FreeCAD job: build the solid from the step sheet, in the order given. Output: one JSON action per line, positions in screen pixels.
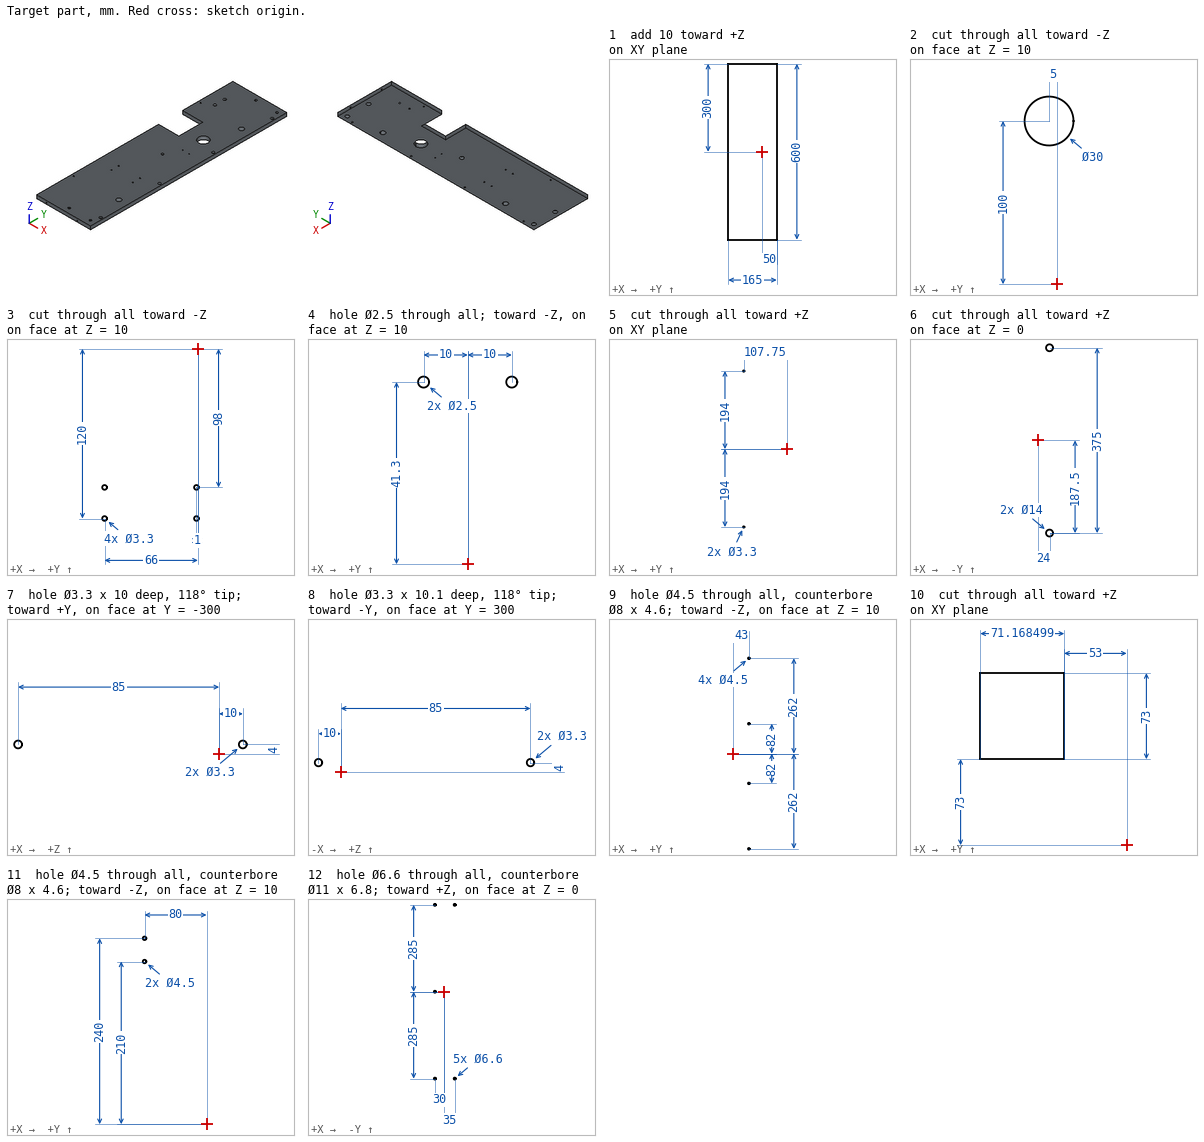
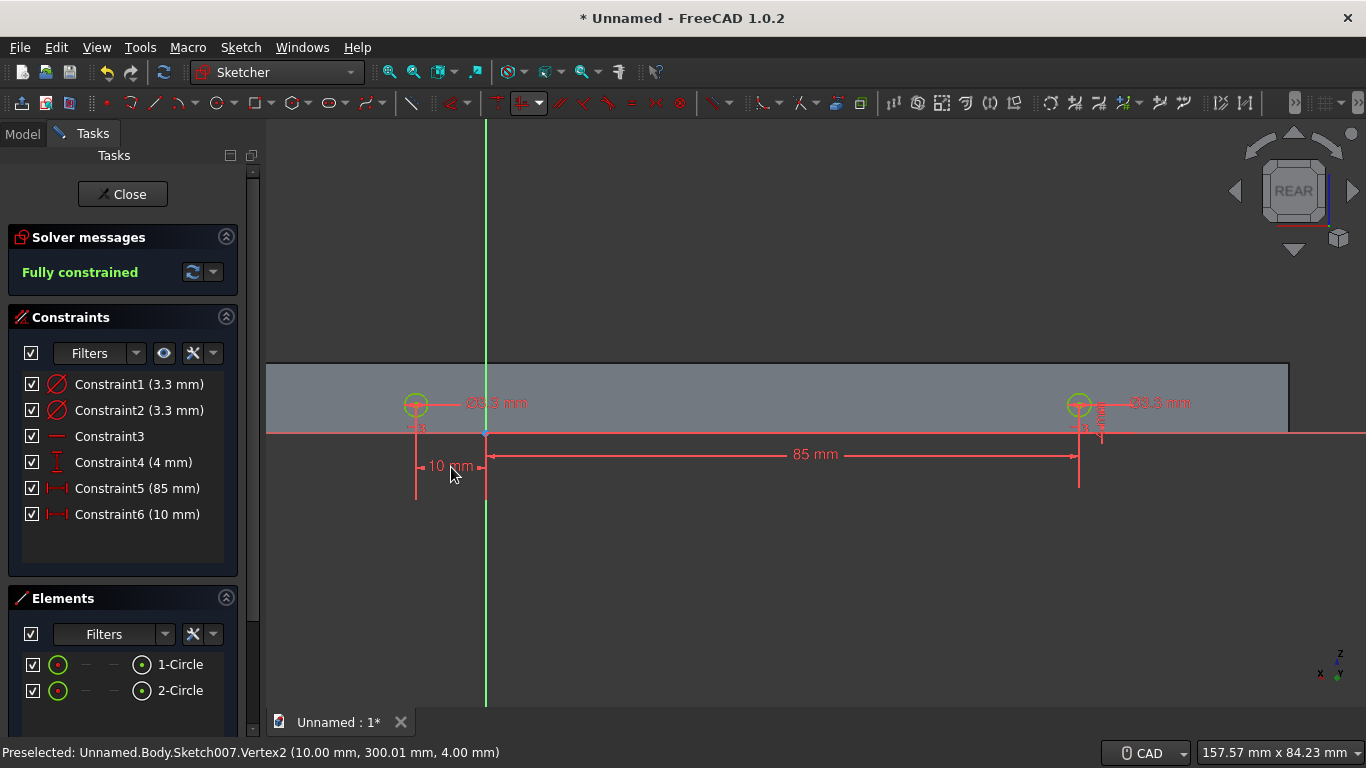
{"action": "left_click", "coordinate": [123, 194]}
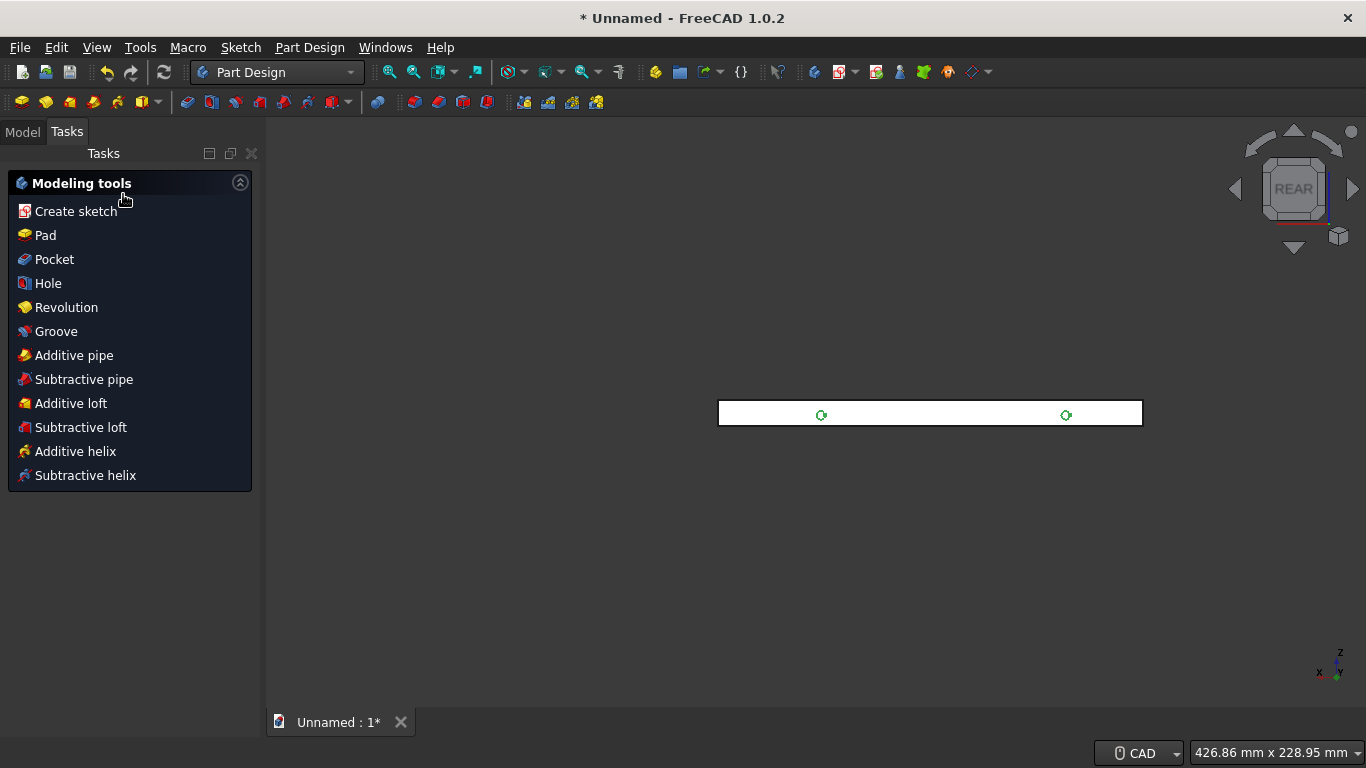
{"action": "left_click", "coordinate": [212, 102]}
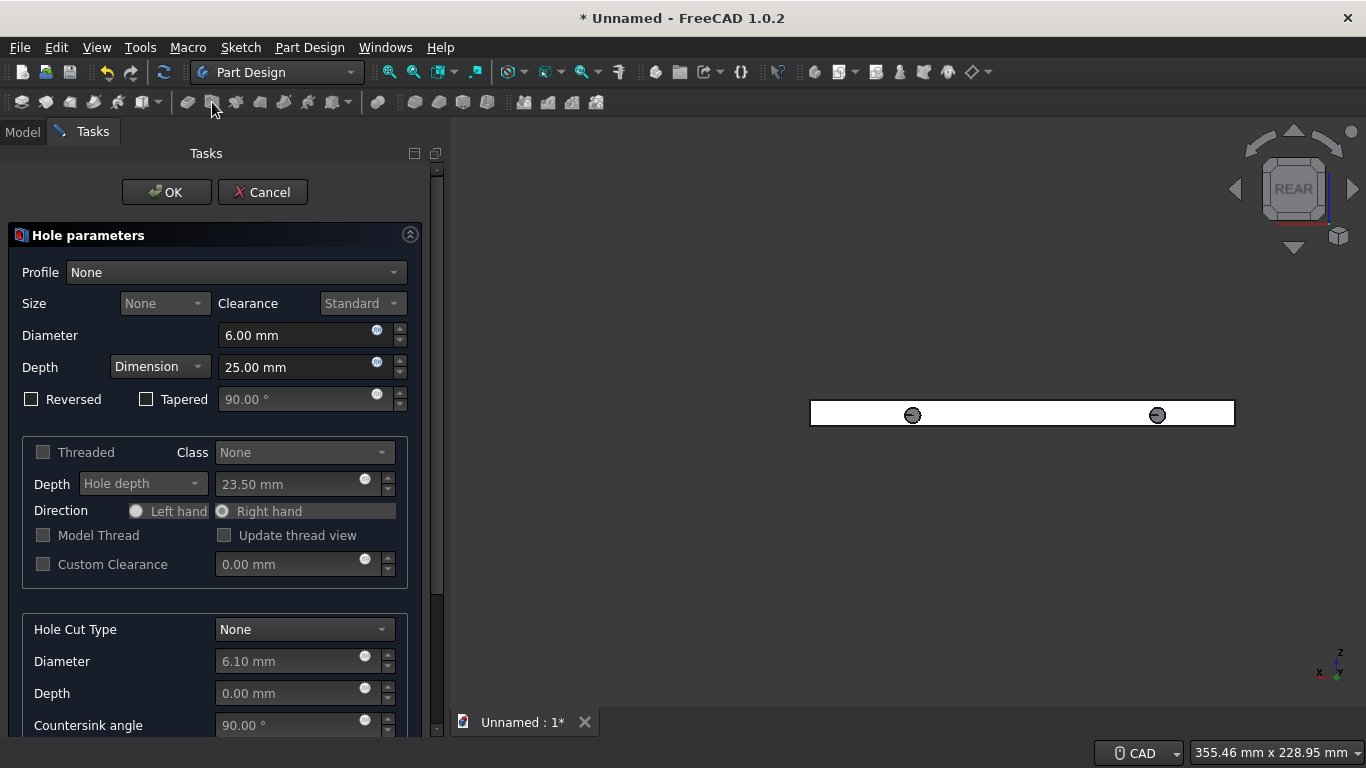
{"action": "triple_click", "coordinate": [305, 335]}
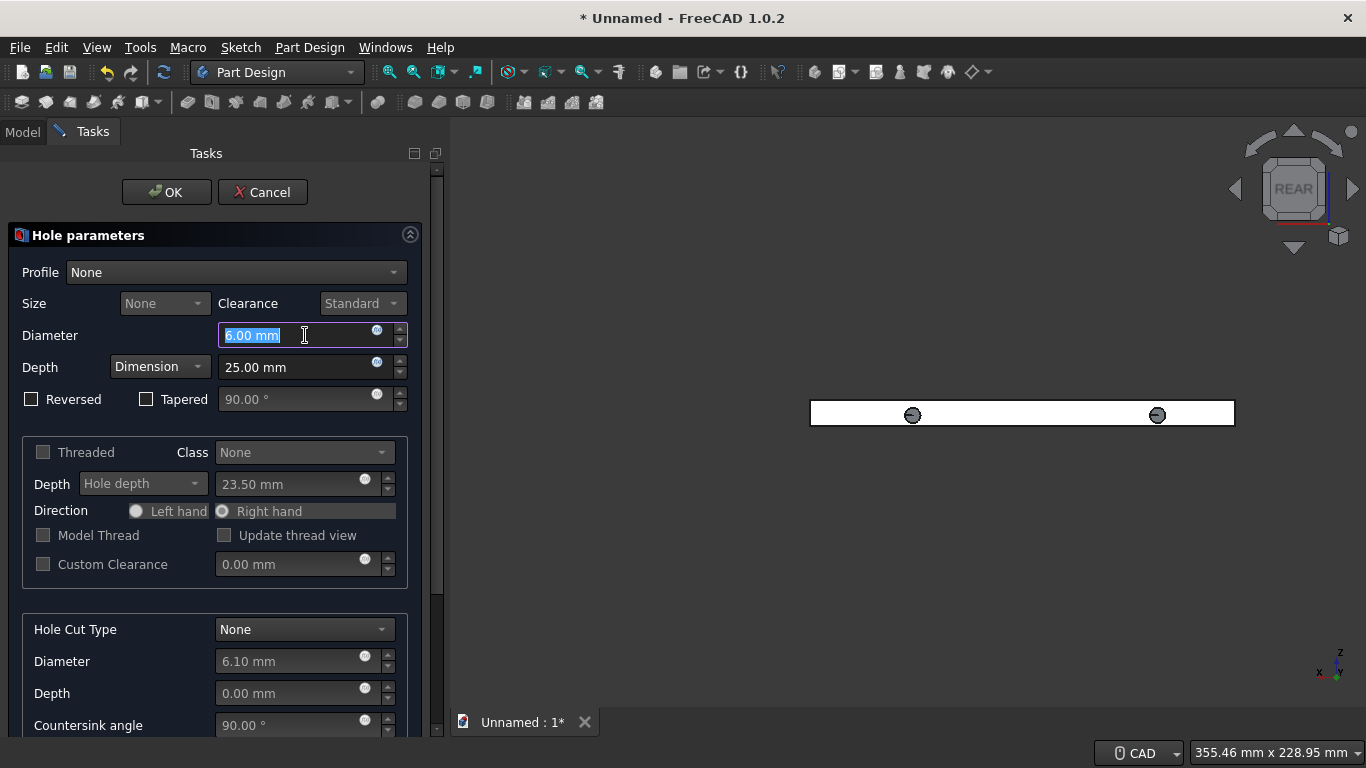
{"action": "type", "text": "3.3"}
{"action": "key", "text": "Tab"}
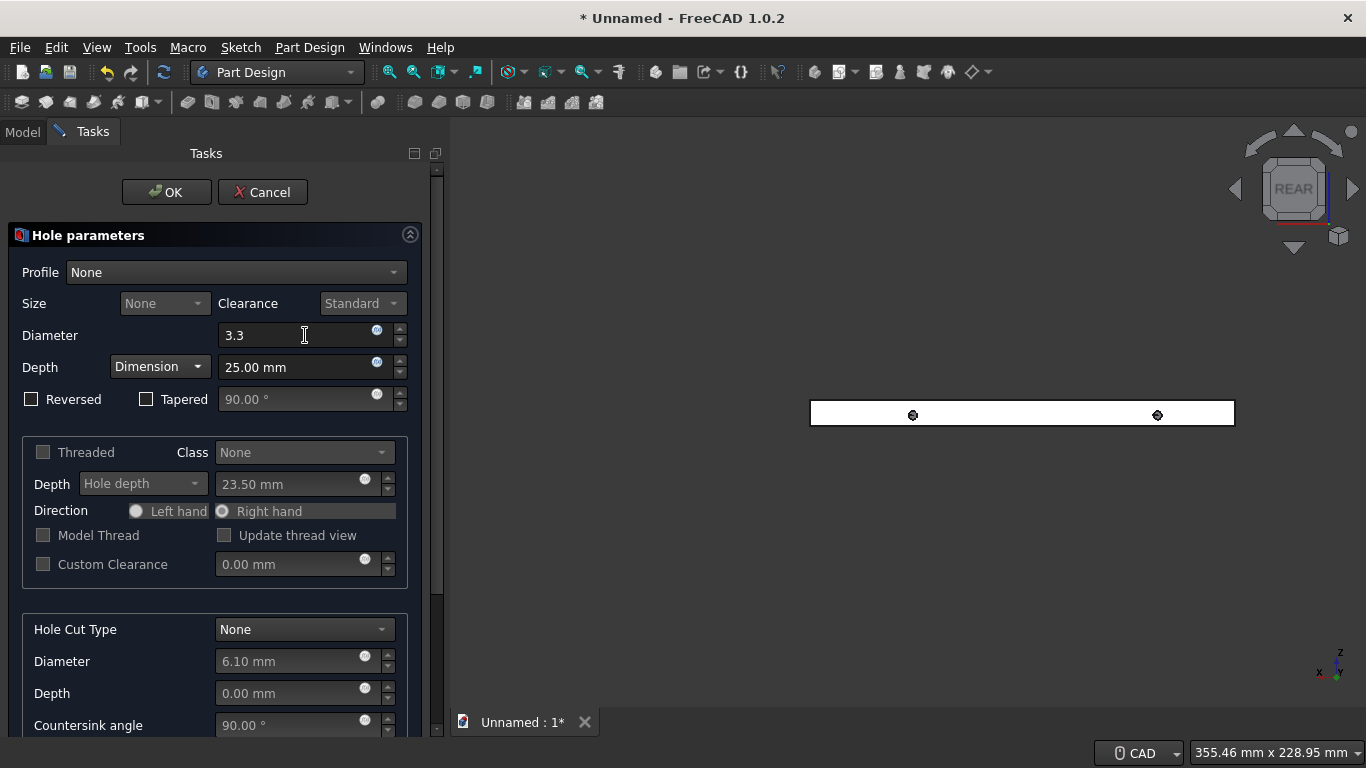
{"action": "triple_click", "coordinate": [305, 367]}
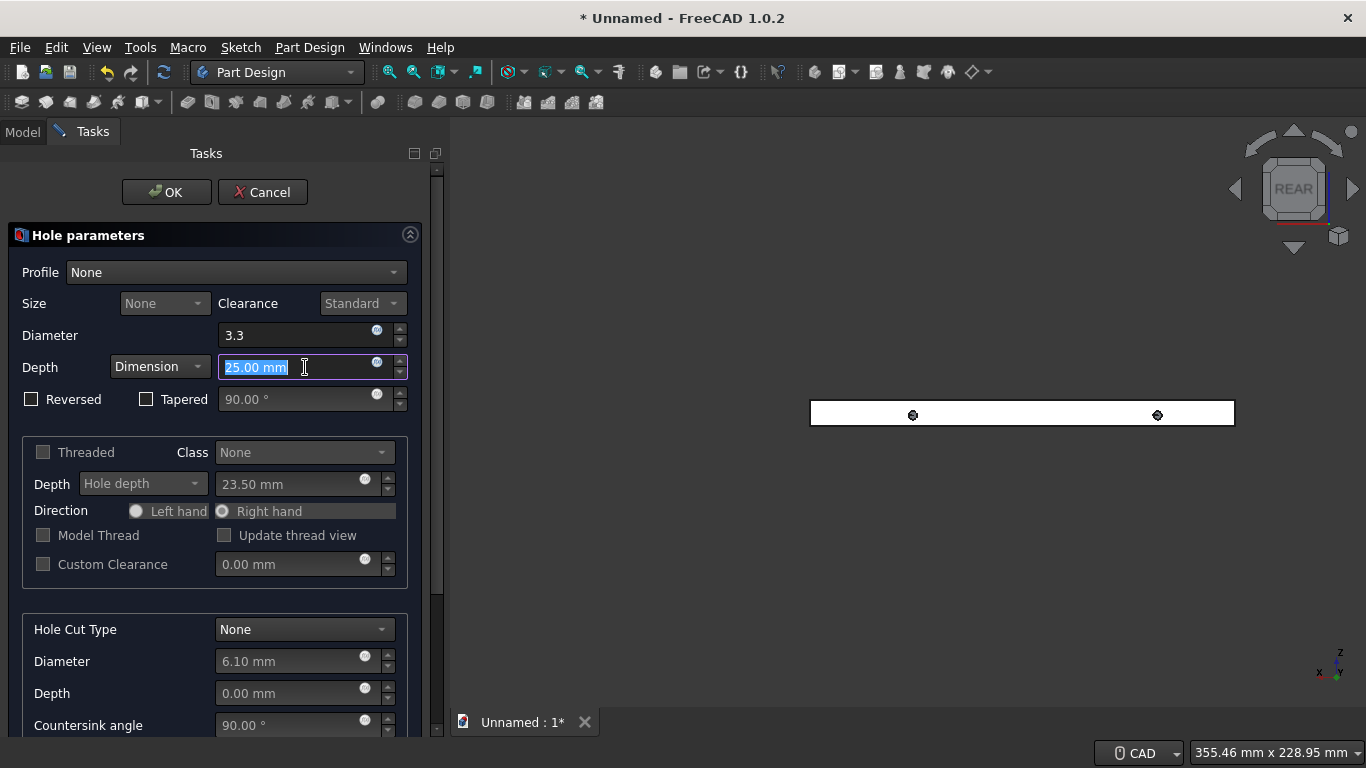
{"action": "type", "text": "10.1"}
{"action": "key", "text": "Tab"}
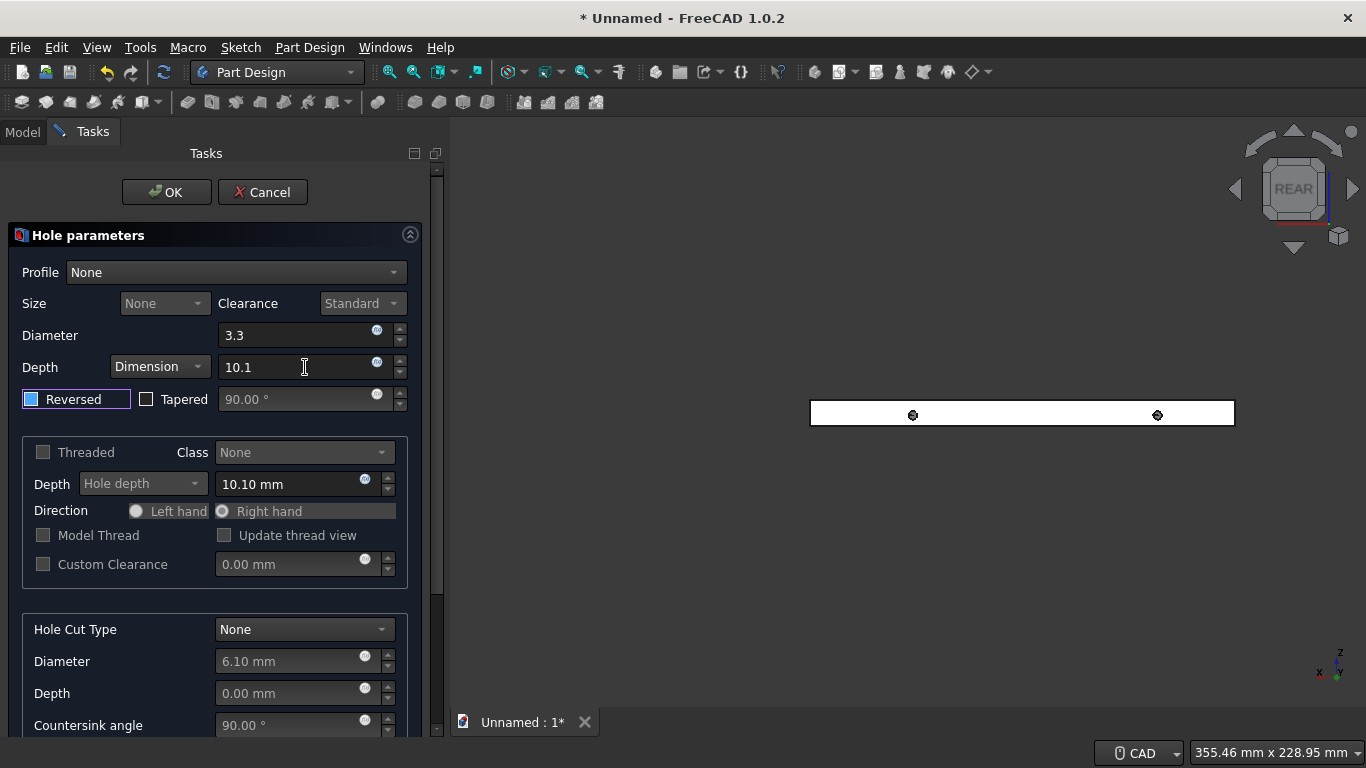
{"action": "left_click", "coordinate": [167, 192]}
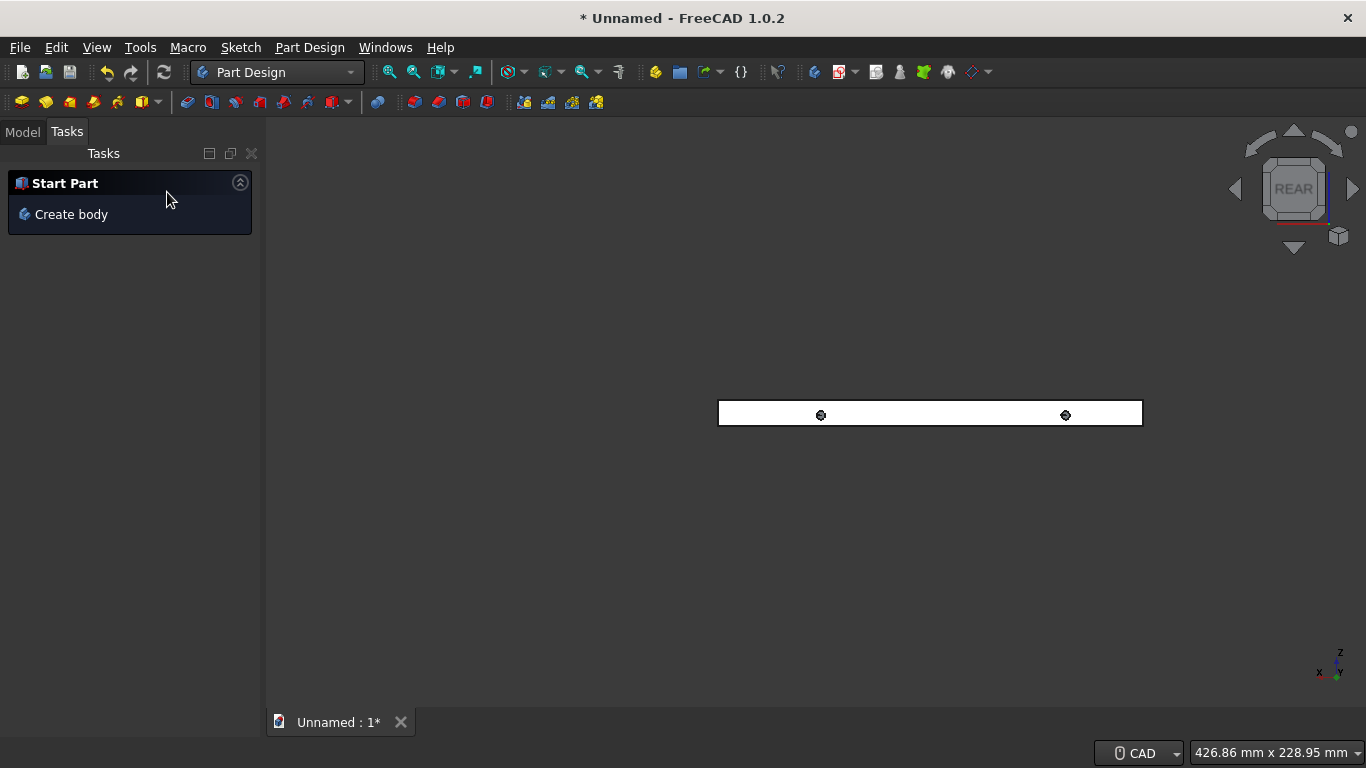
{"action": "left_click", "coordinate": [390, 72]}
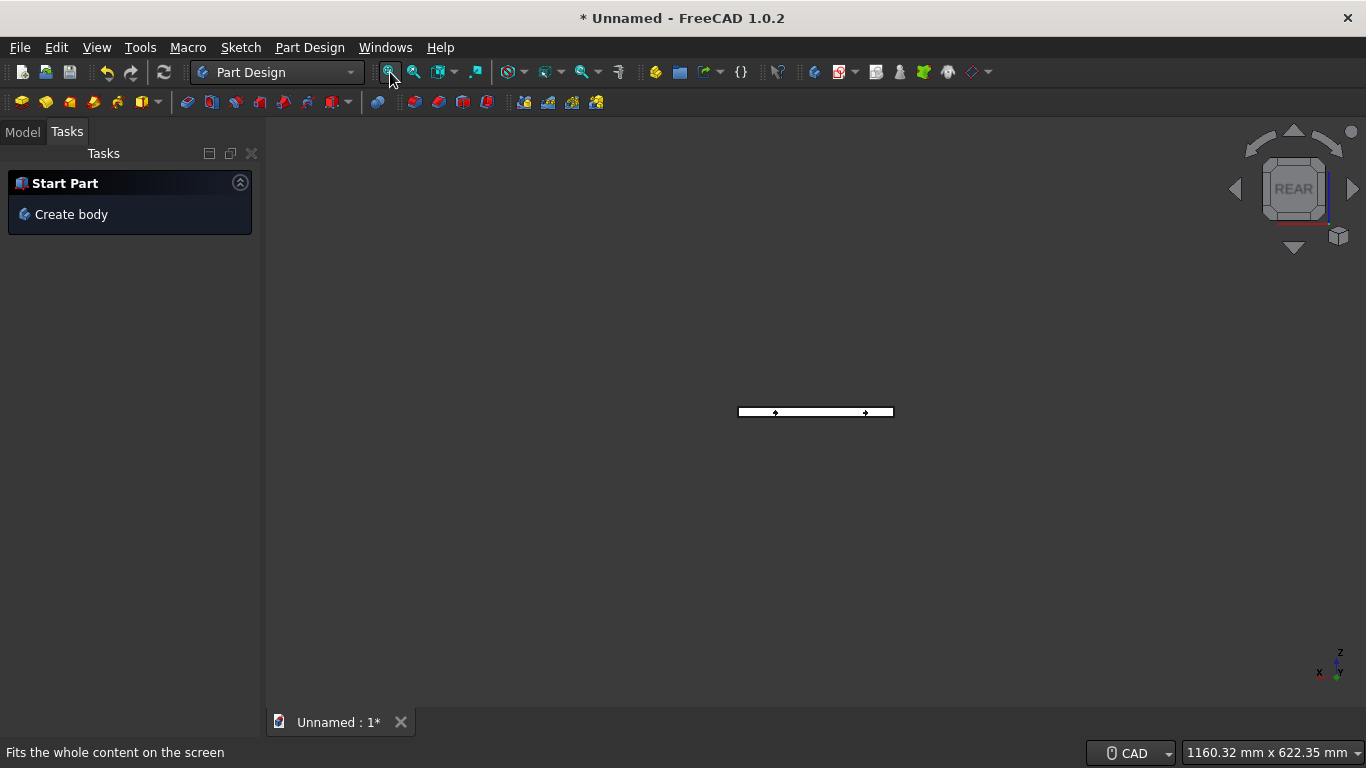
{"action": "key", "text": "0"}